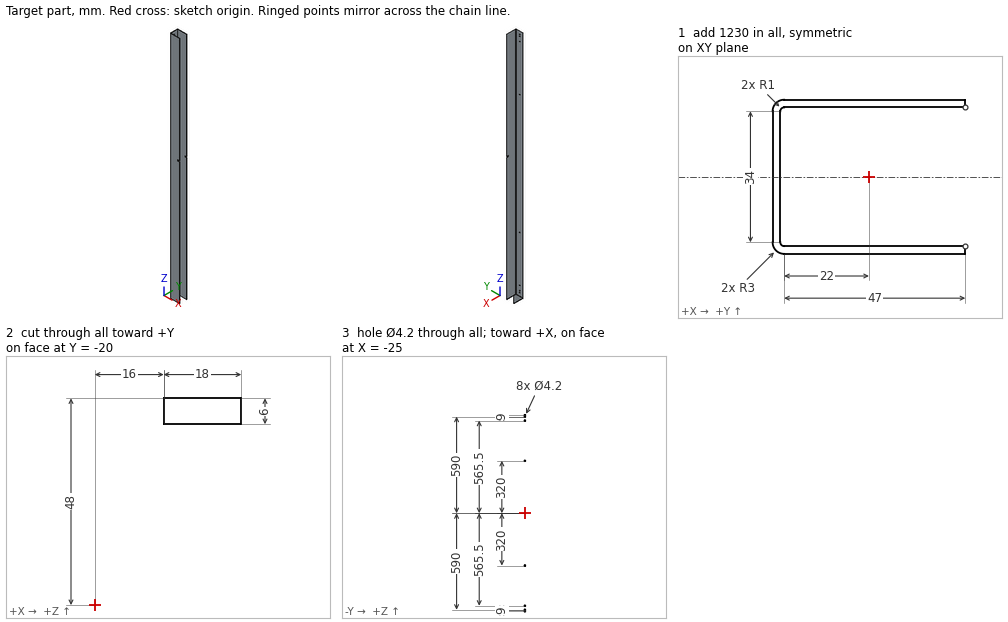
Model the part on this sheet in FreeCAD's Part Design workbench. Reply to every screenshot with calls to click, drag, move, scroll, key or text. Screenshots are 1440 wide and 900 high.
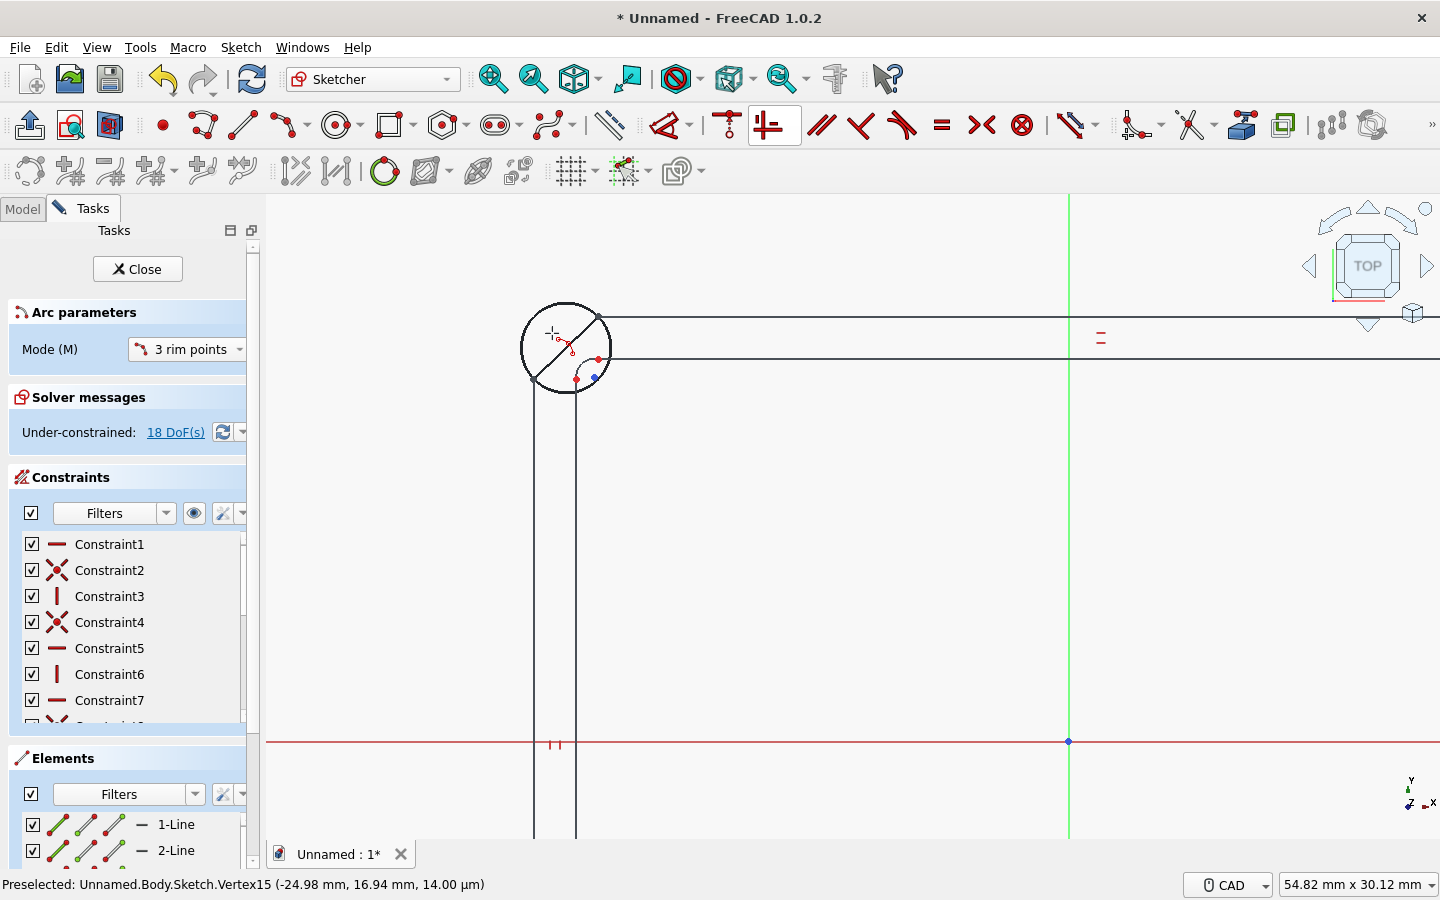
click(552, 332)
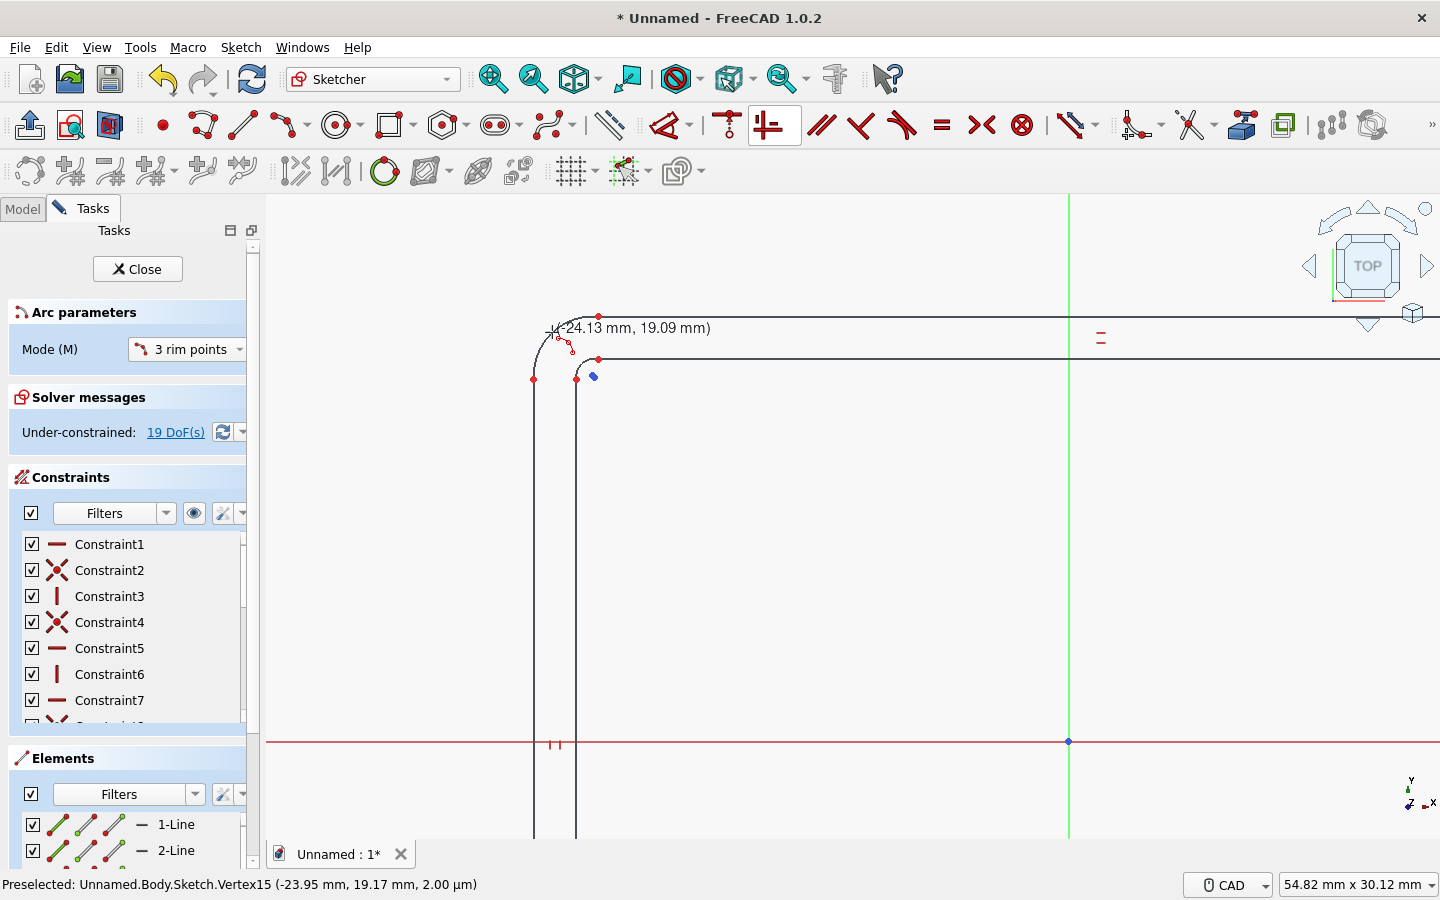
scroll(553, 333, down, 4)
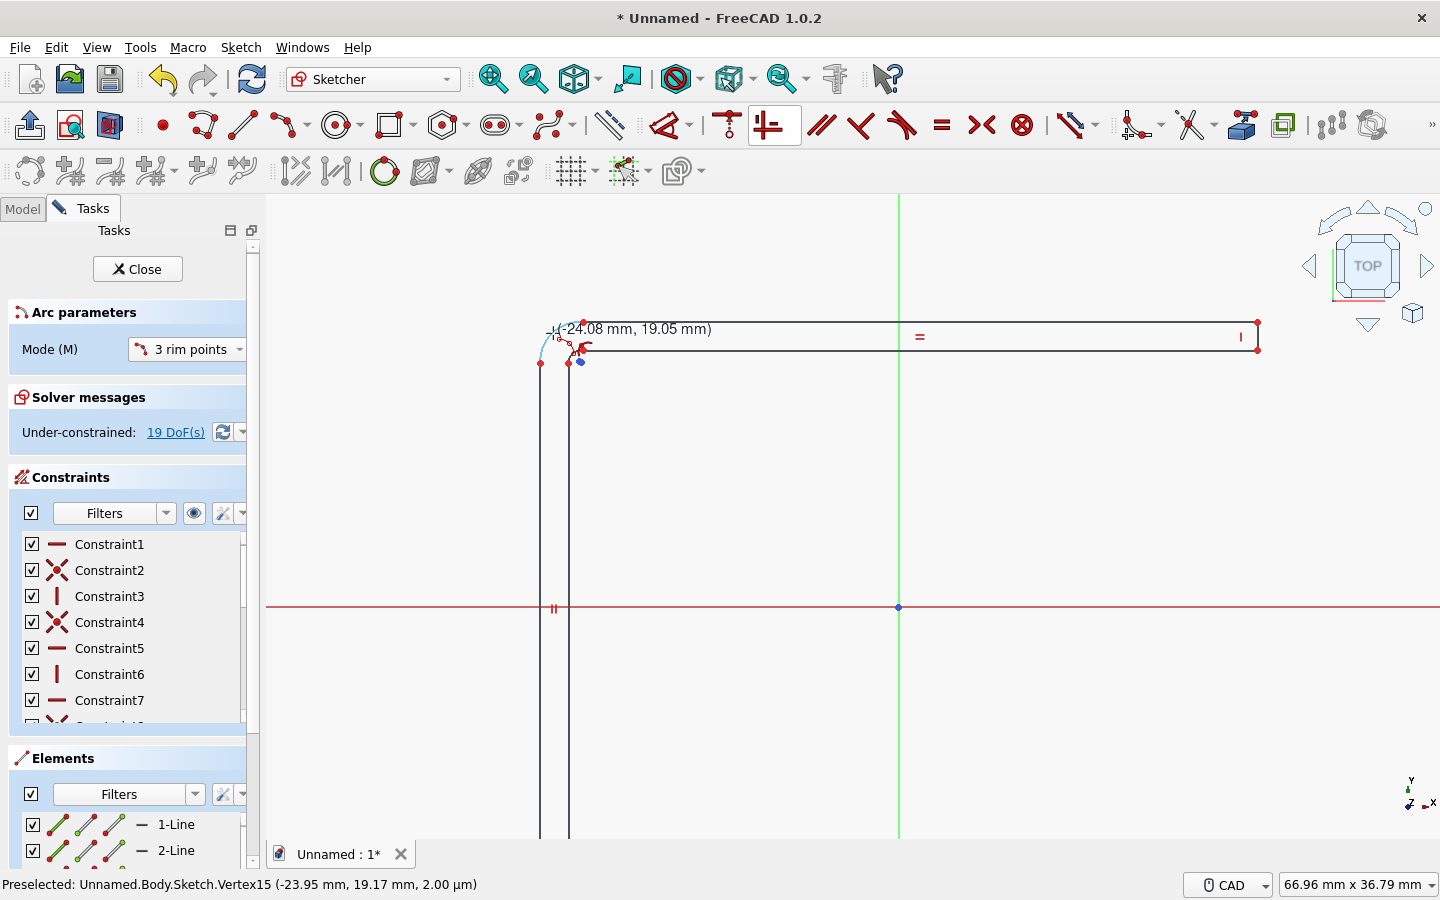
click(545, 682)
click(574, 710)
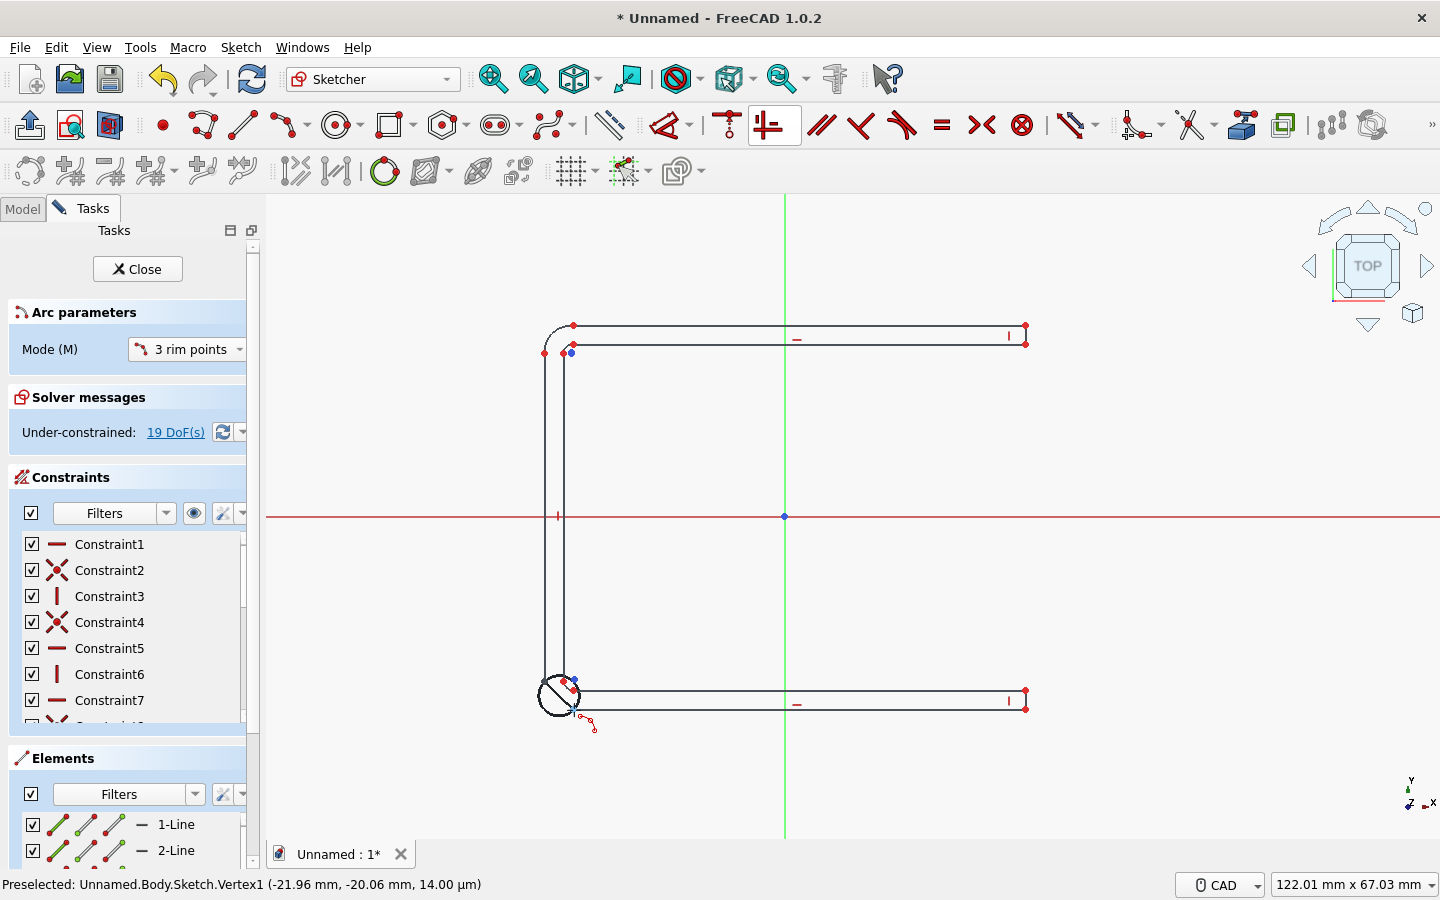
scroll(553, 701, up, 4)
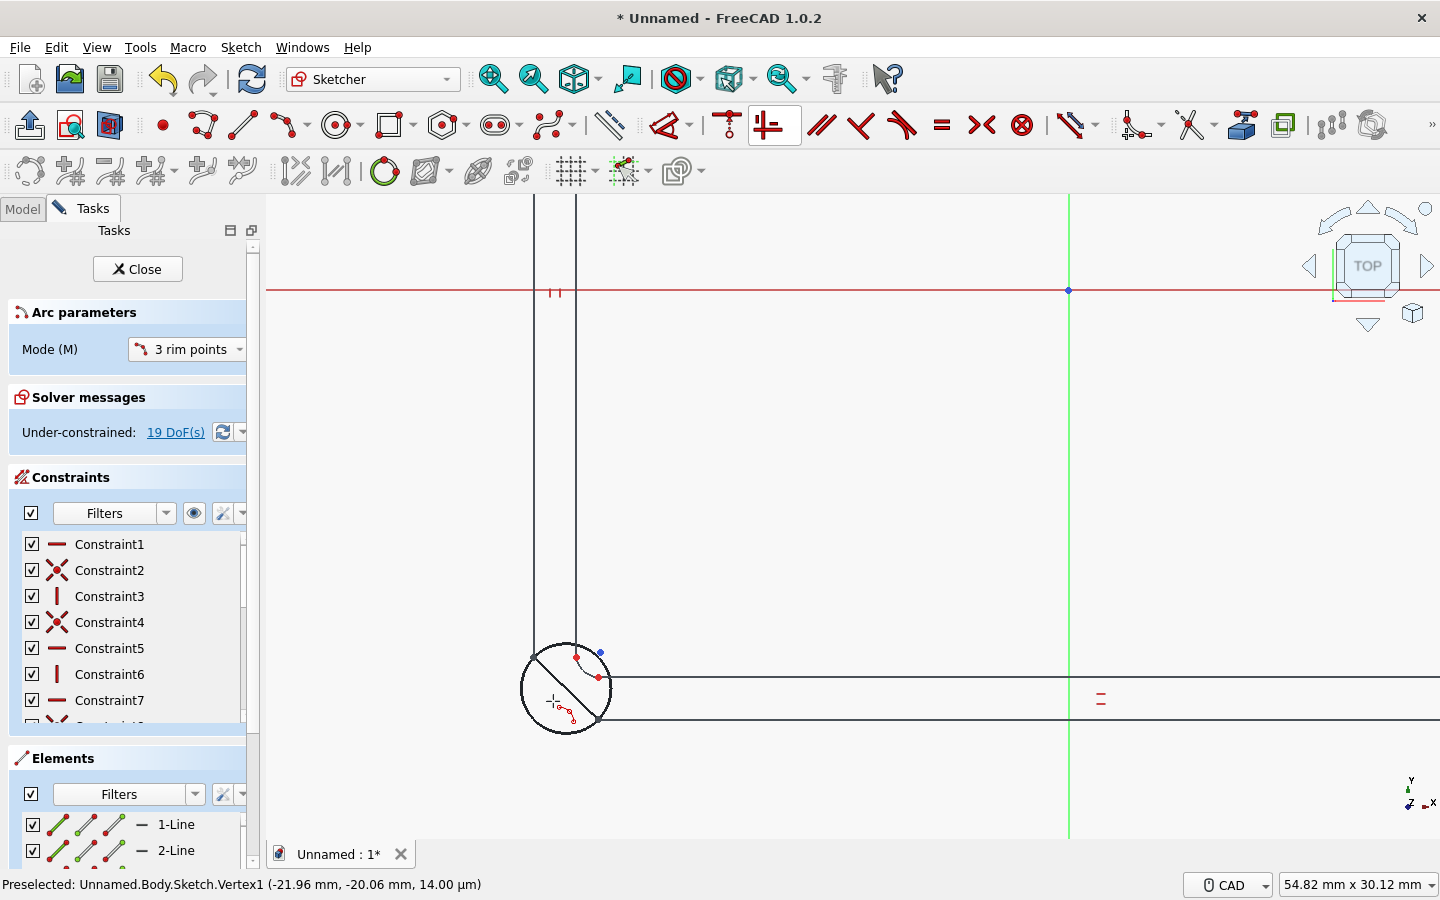
click(552, 700)
key(Escape)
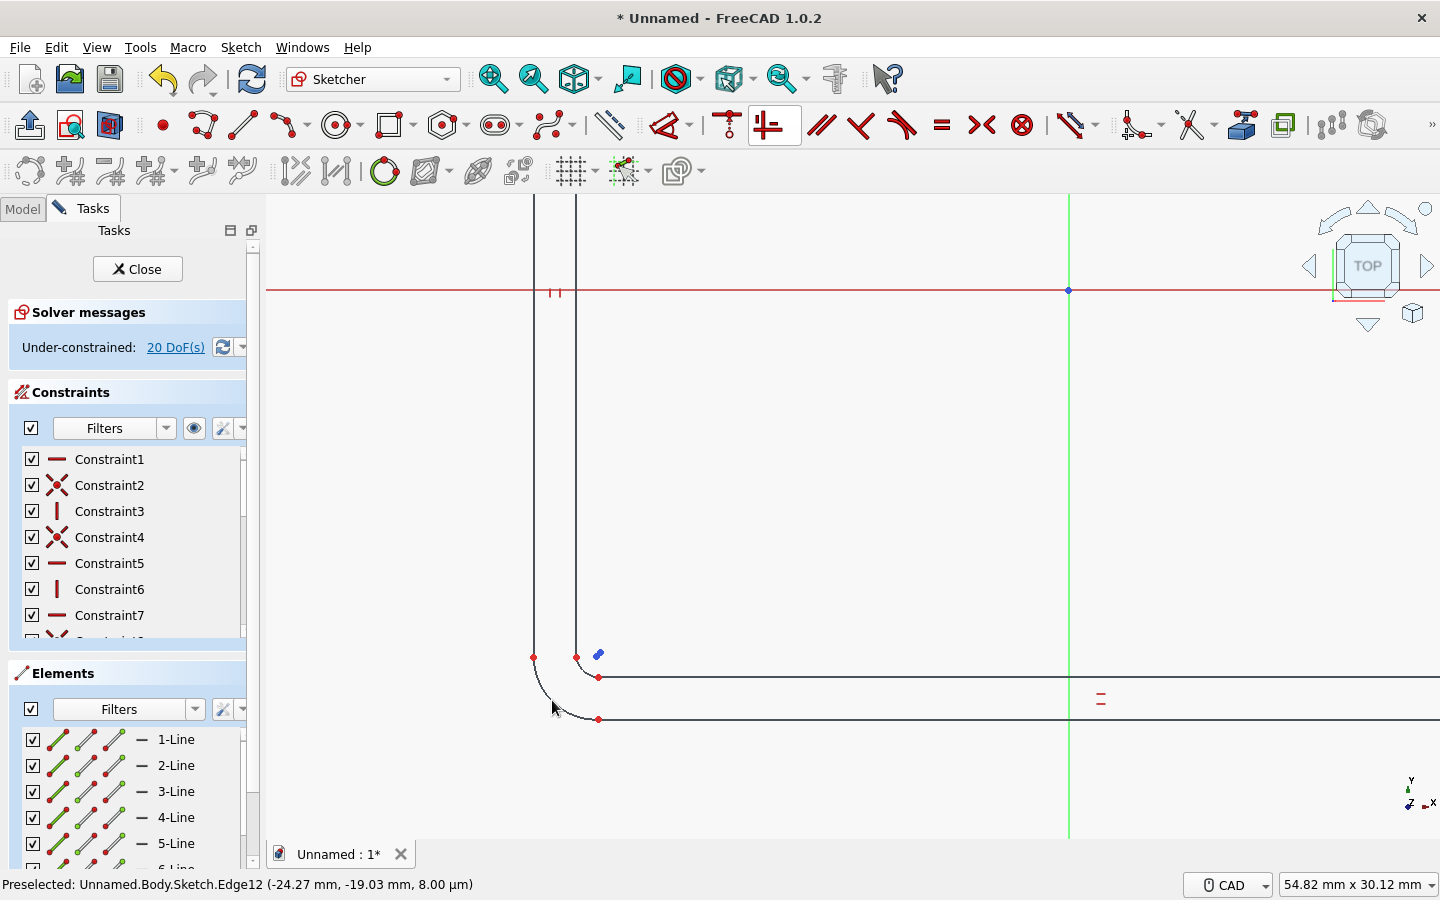
click(900, 720)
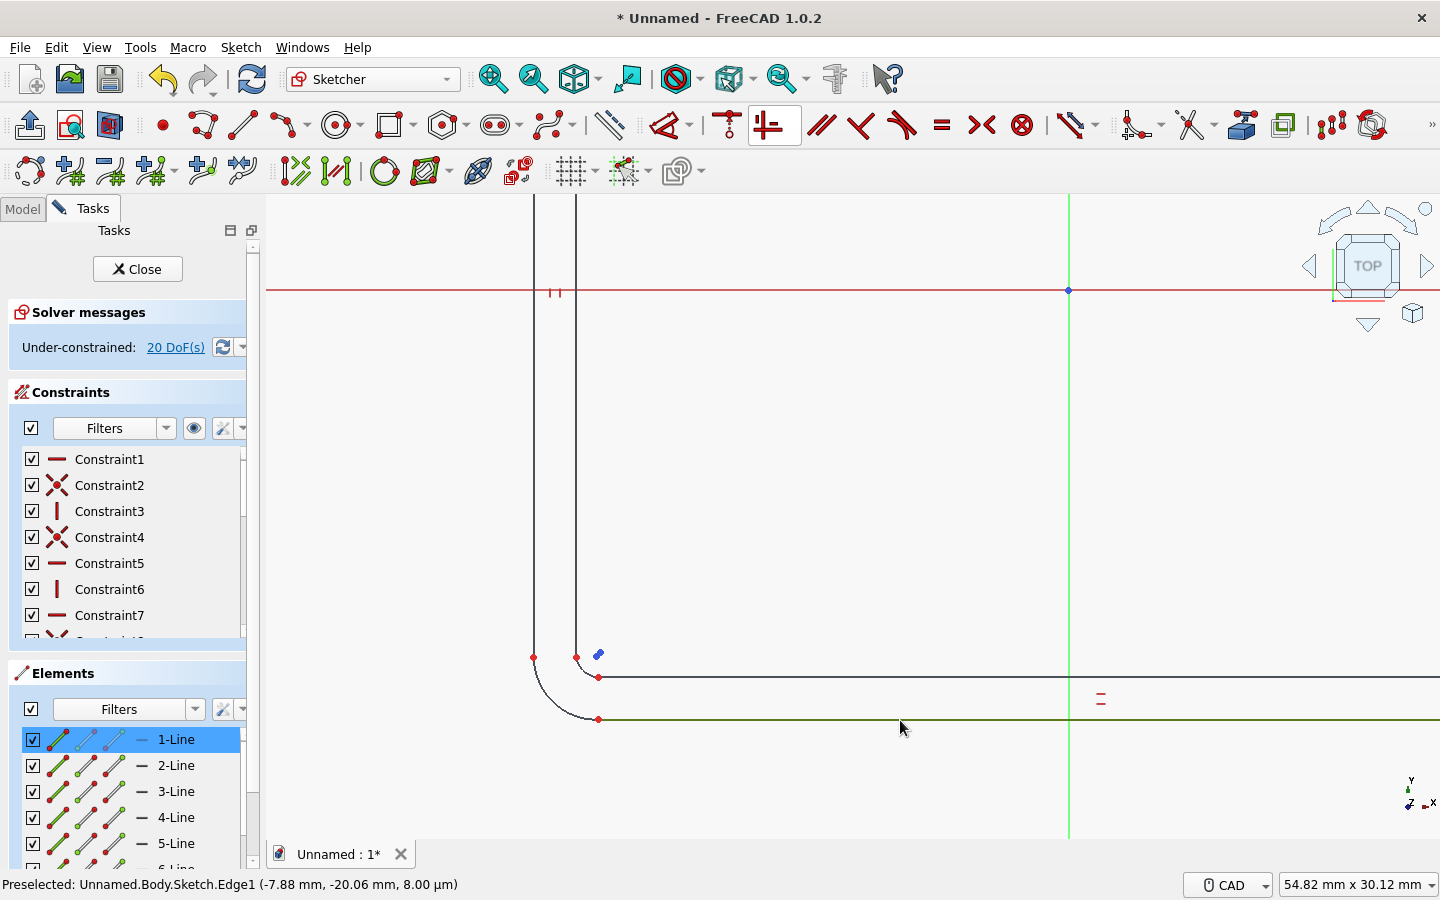
click(541, 686)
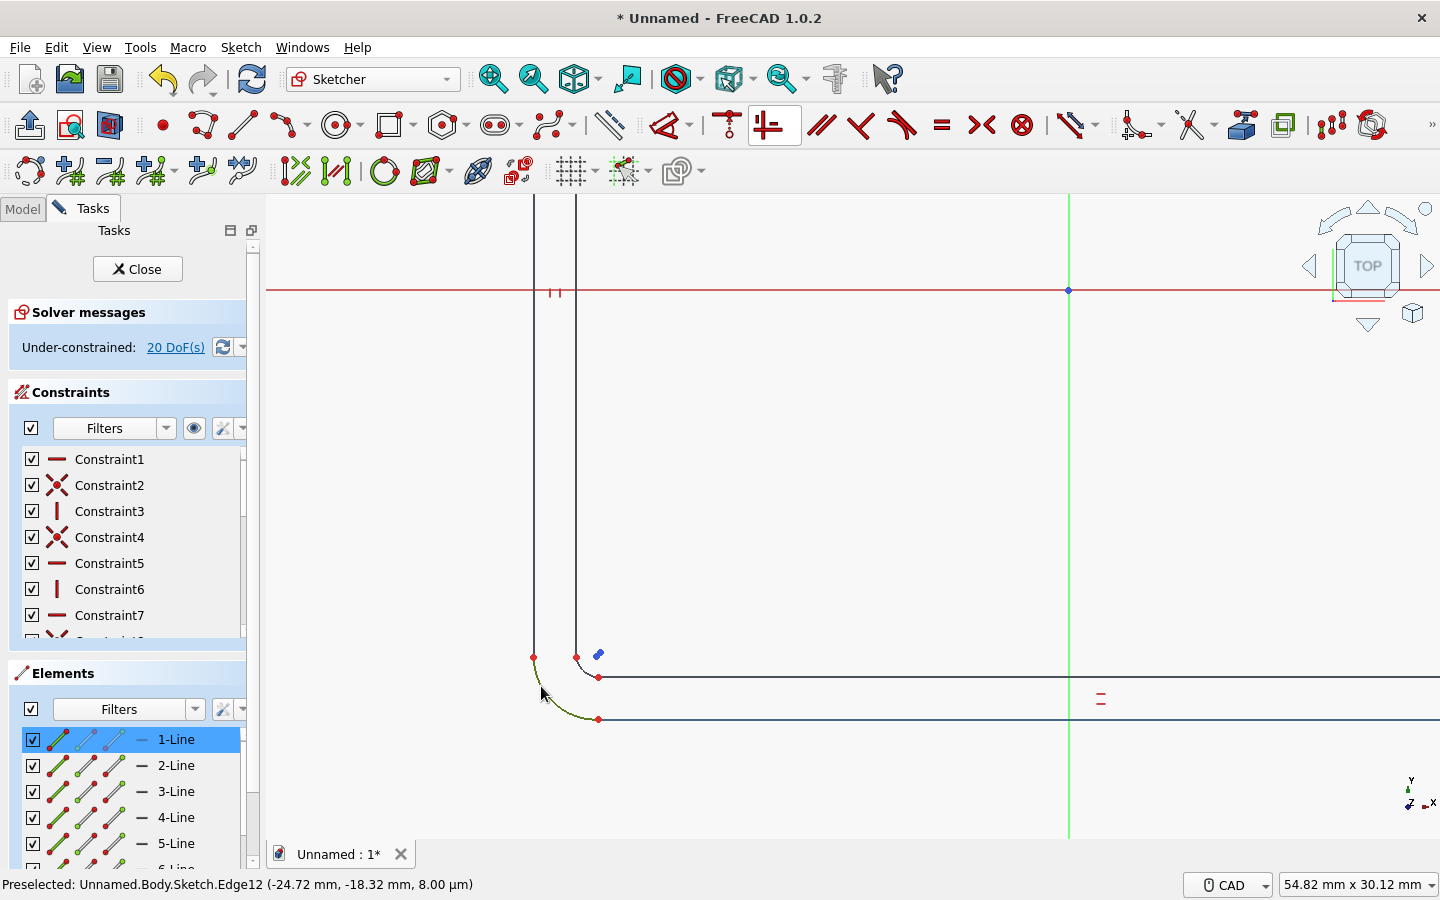
key(t)